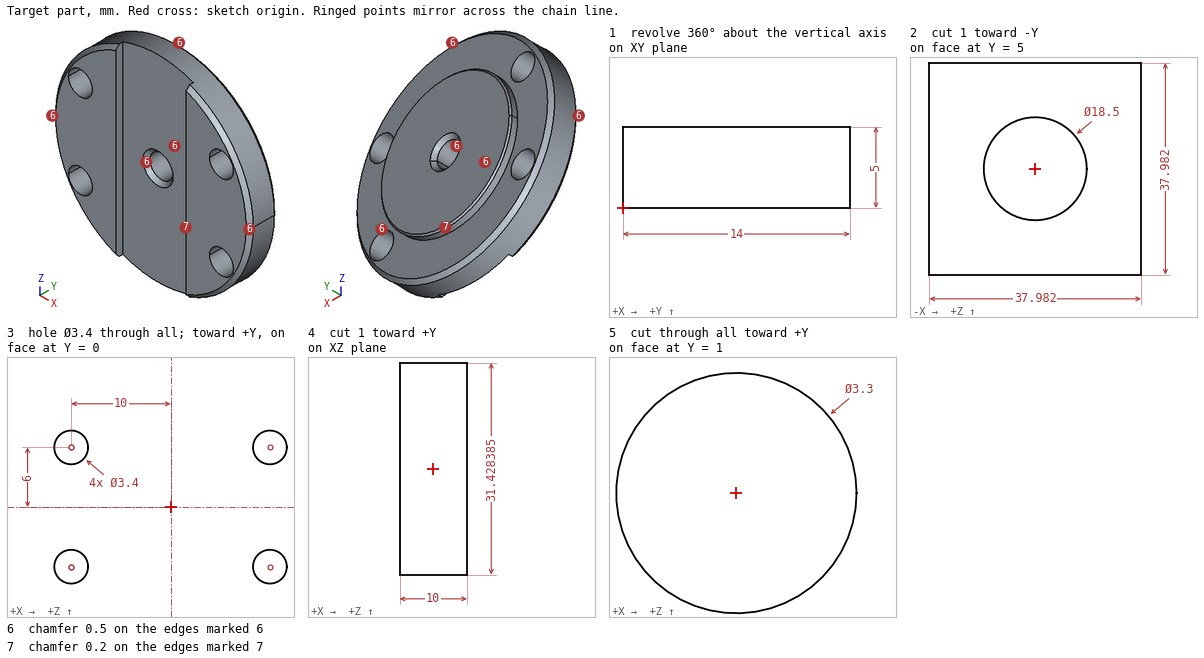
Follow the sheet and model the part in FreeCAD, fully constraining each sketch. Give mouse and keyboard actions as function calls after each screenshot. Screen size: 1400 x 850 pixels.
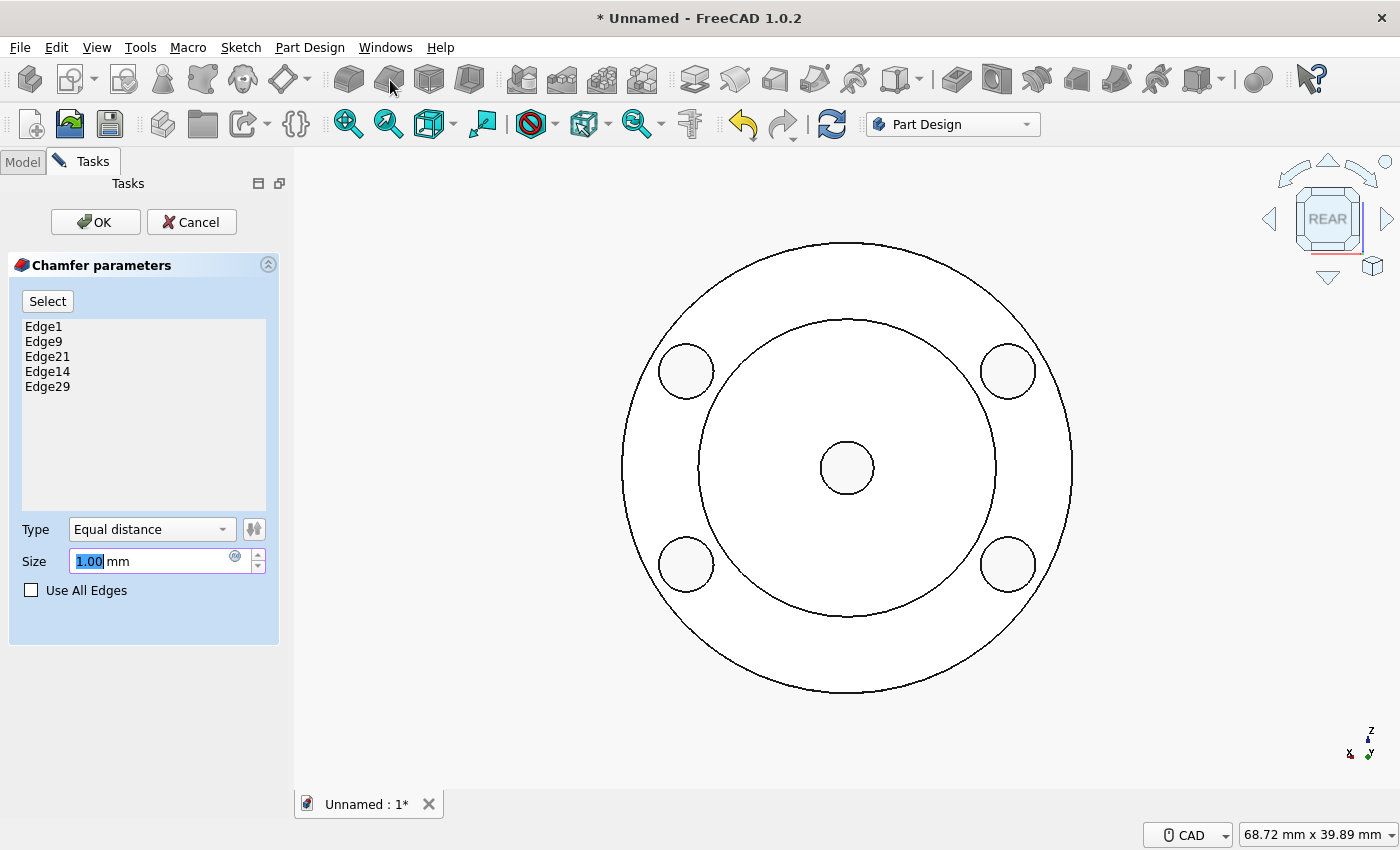
text(0.5)
key(Tab)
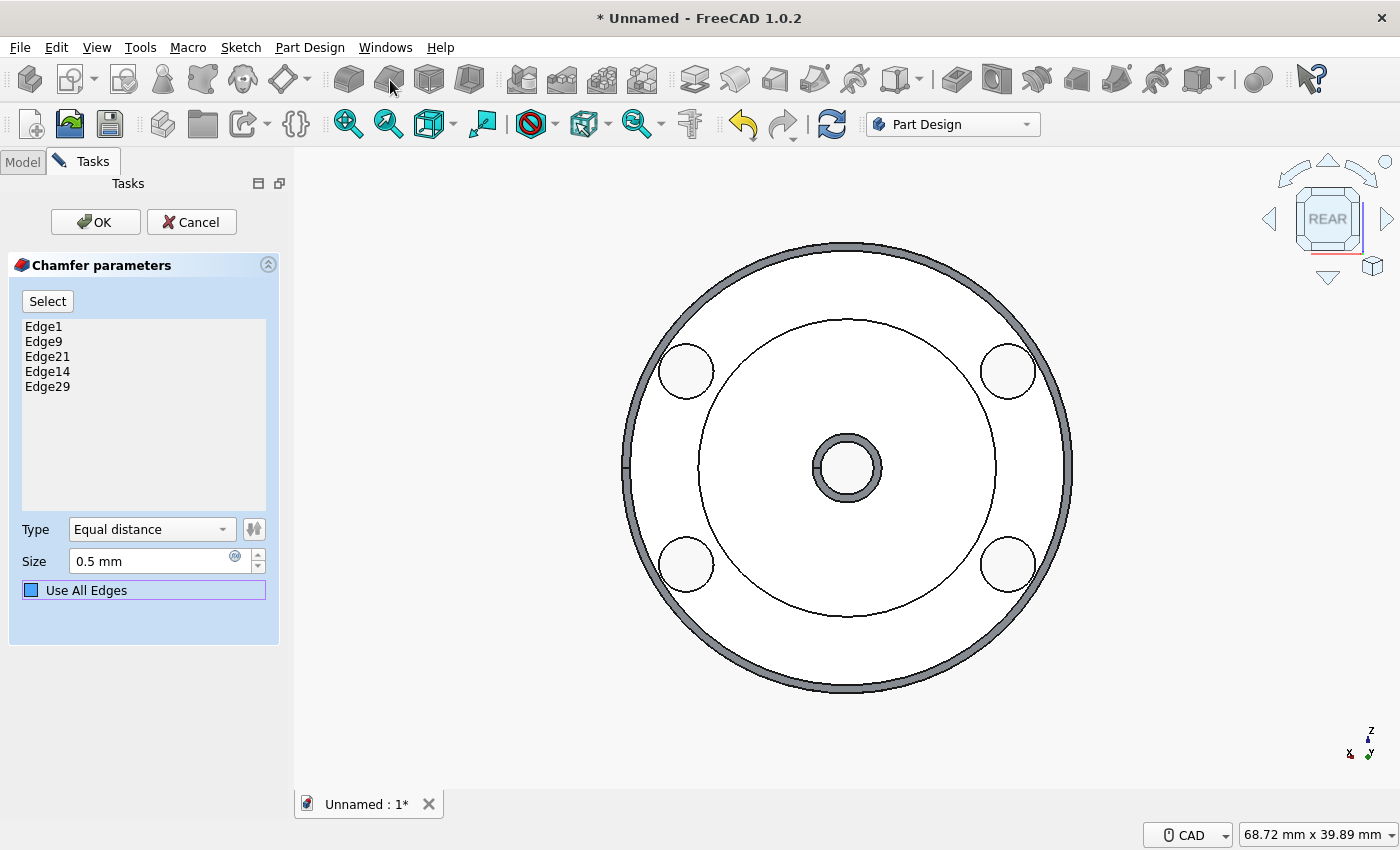
click(96, 222)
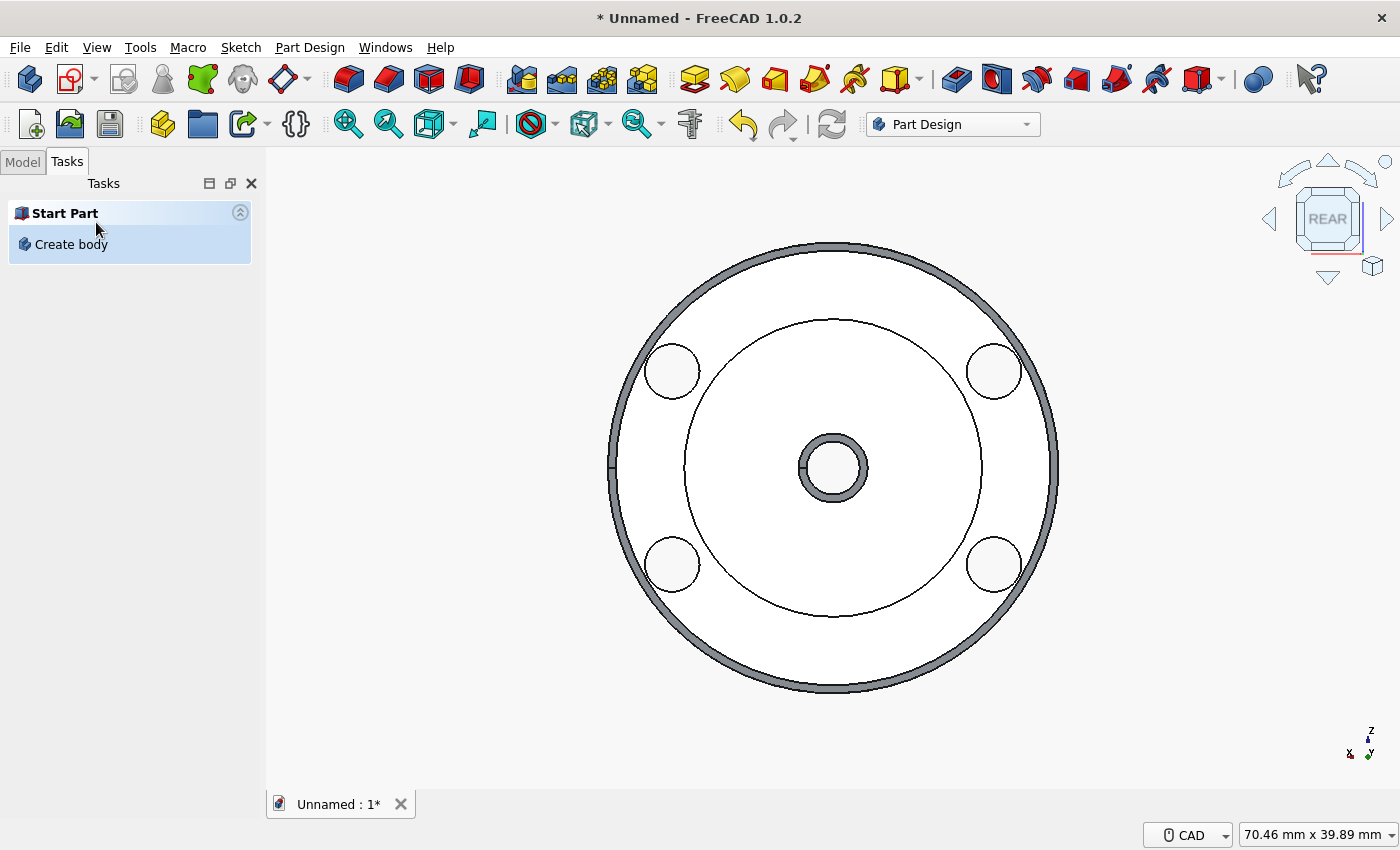
click(684, 467)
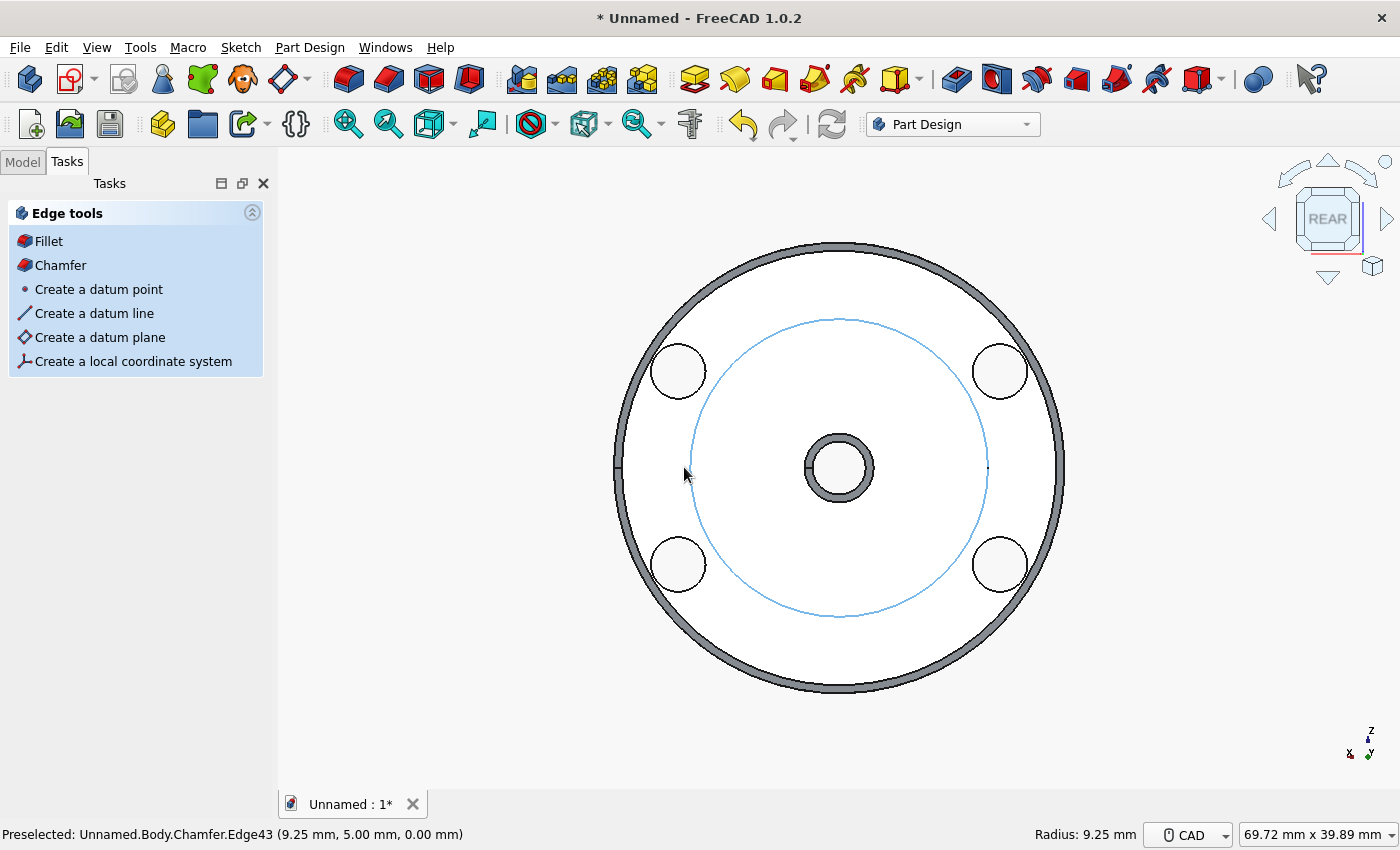
click(390, 80)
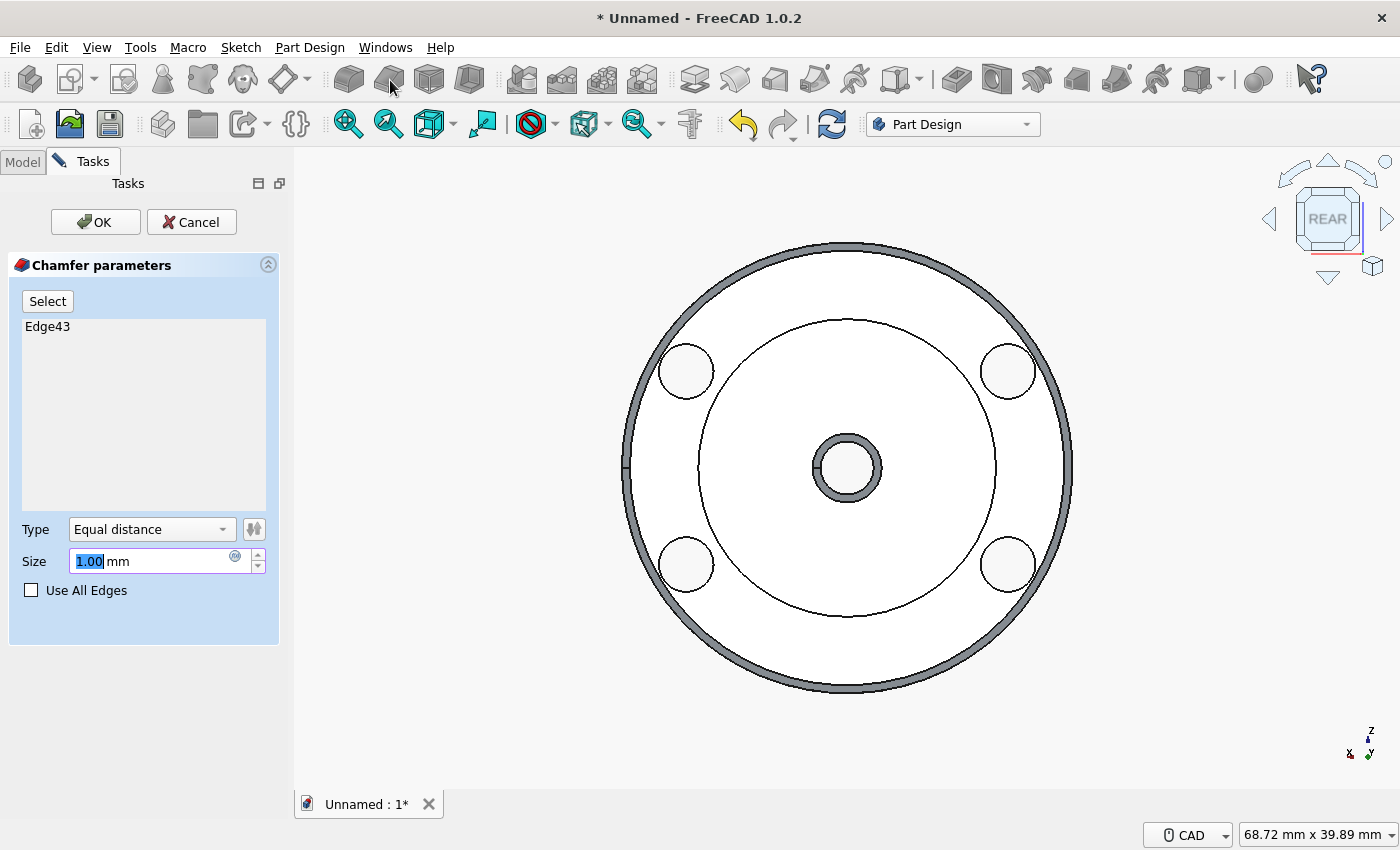
text(0.2)
key(Tab)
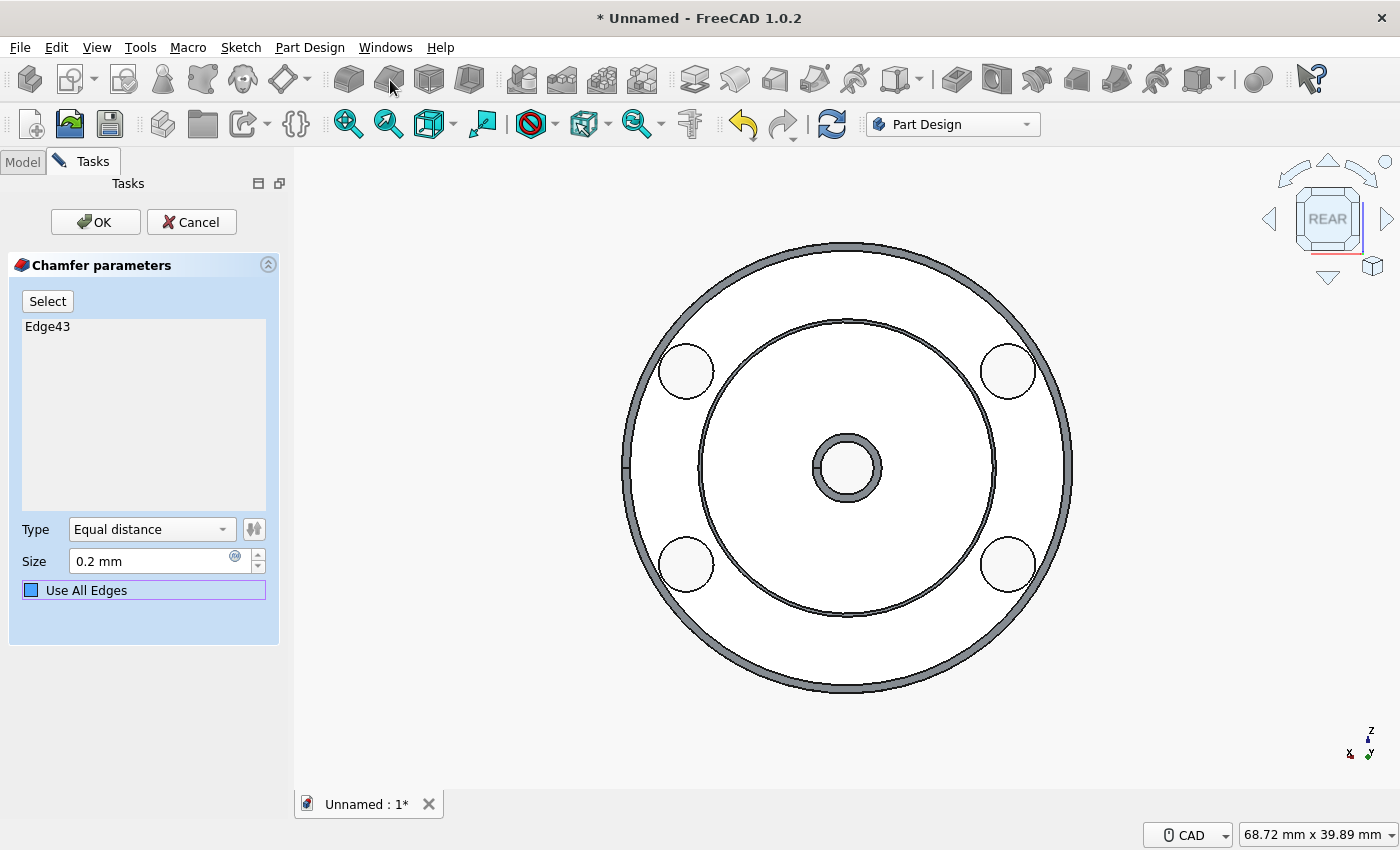
click(96, 222)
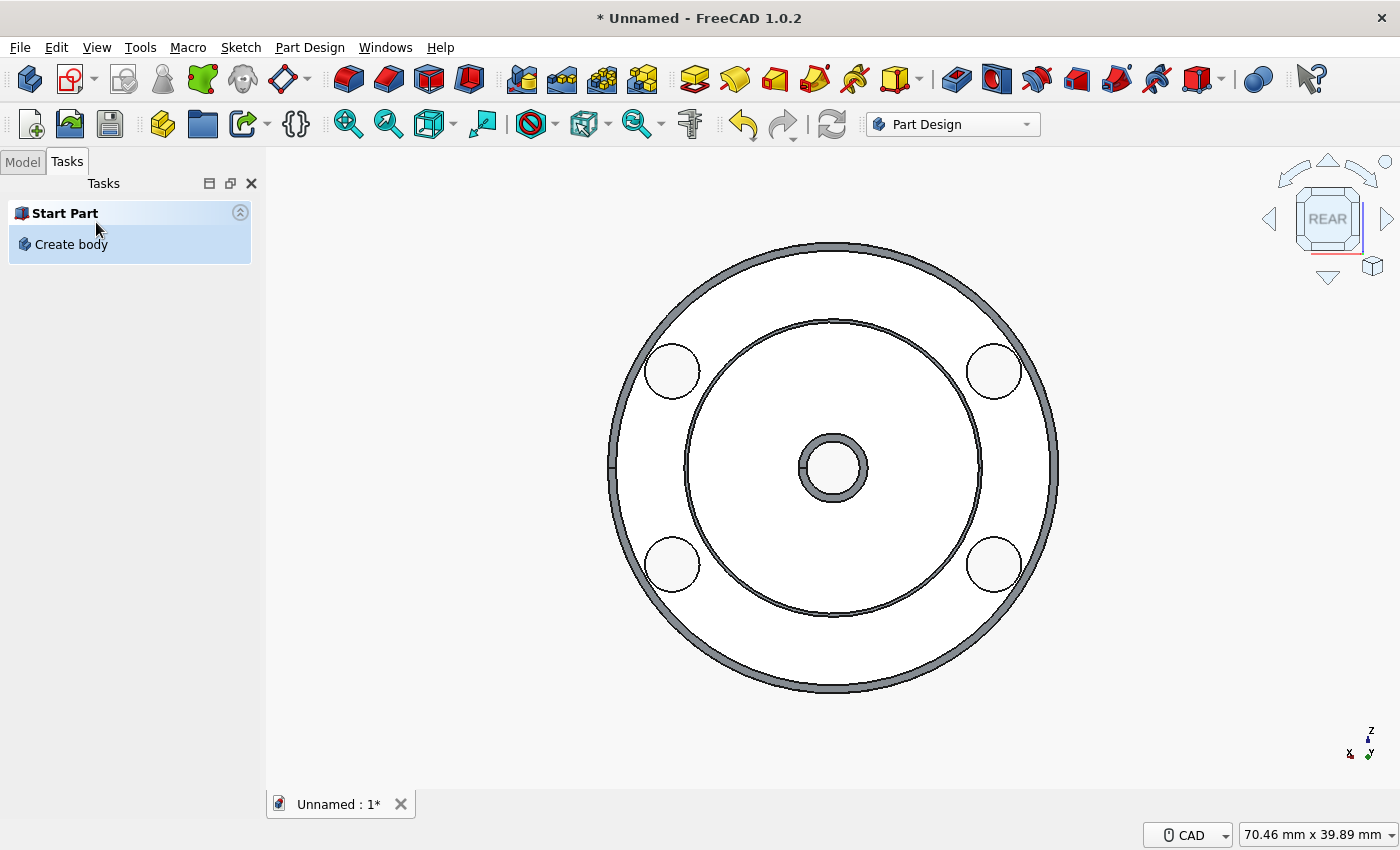
key(0)